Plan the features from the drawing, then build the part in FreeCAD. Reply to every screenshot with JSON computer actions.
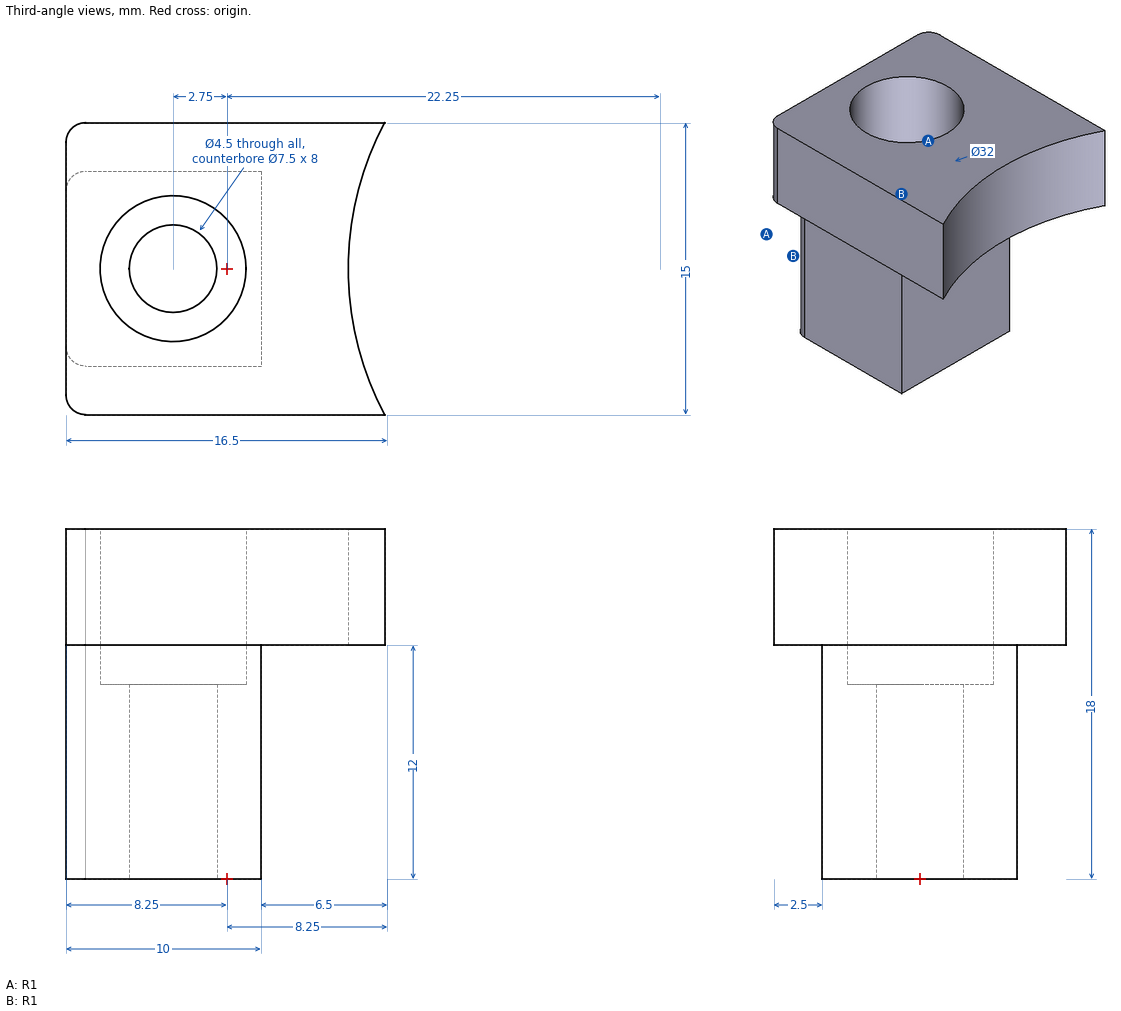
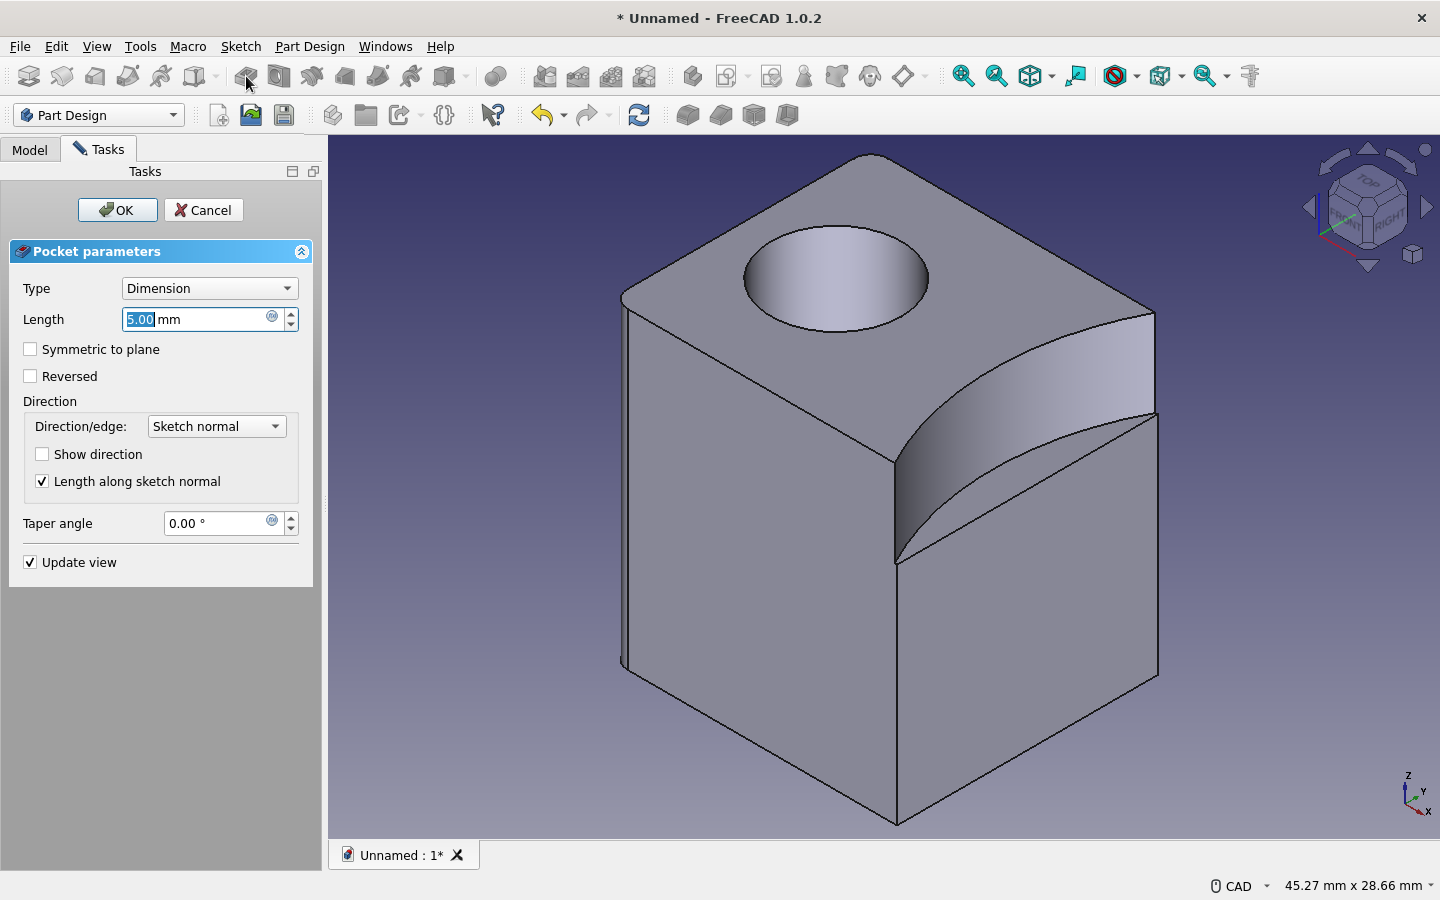
{"action": "left_click", "coordinate": [210, 288]}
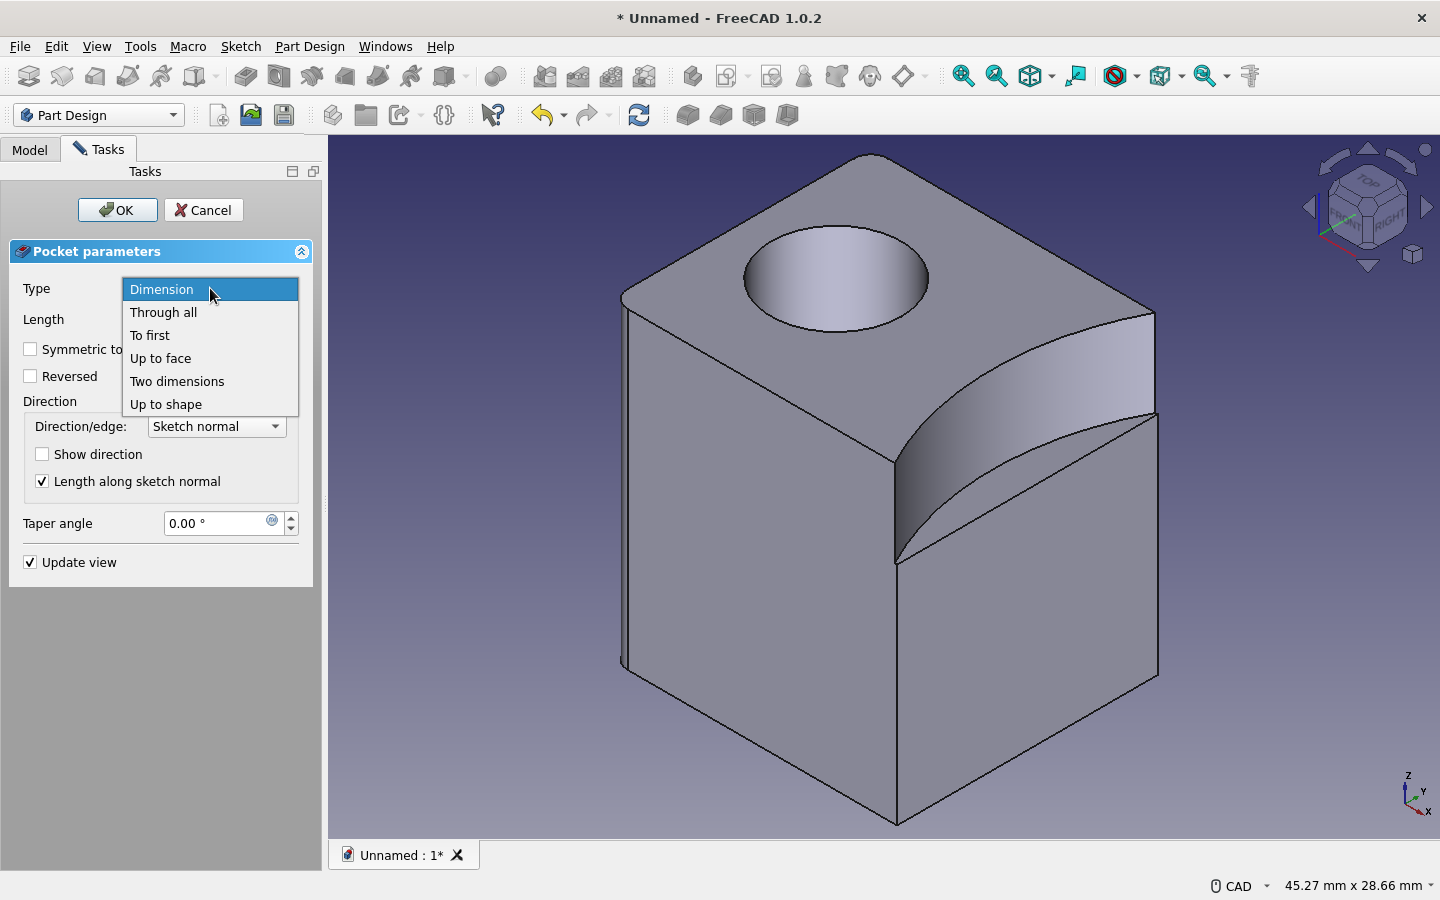
{"action": "left_click", "coordinate": [208, 312]}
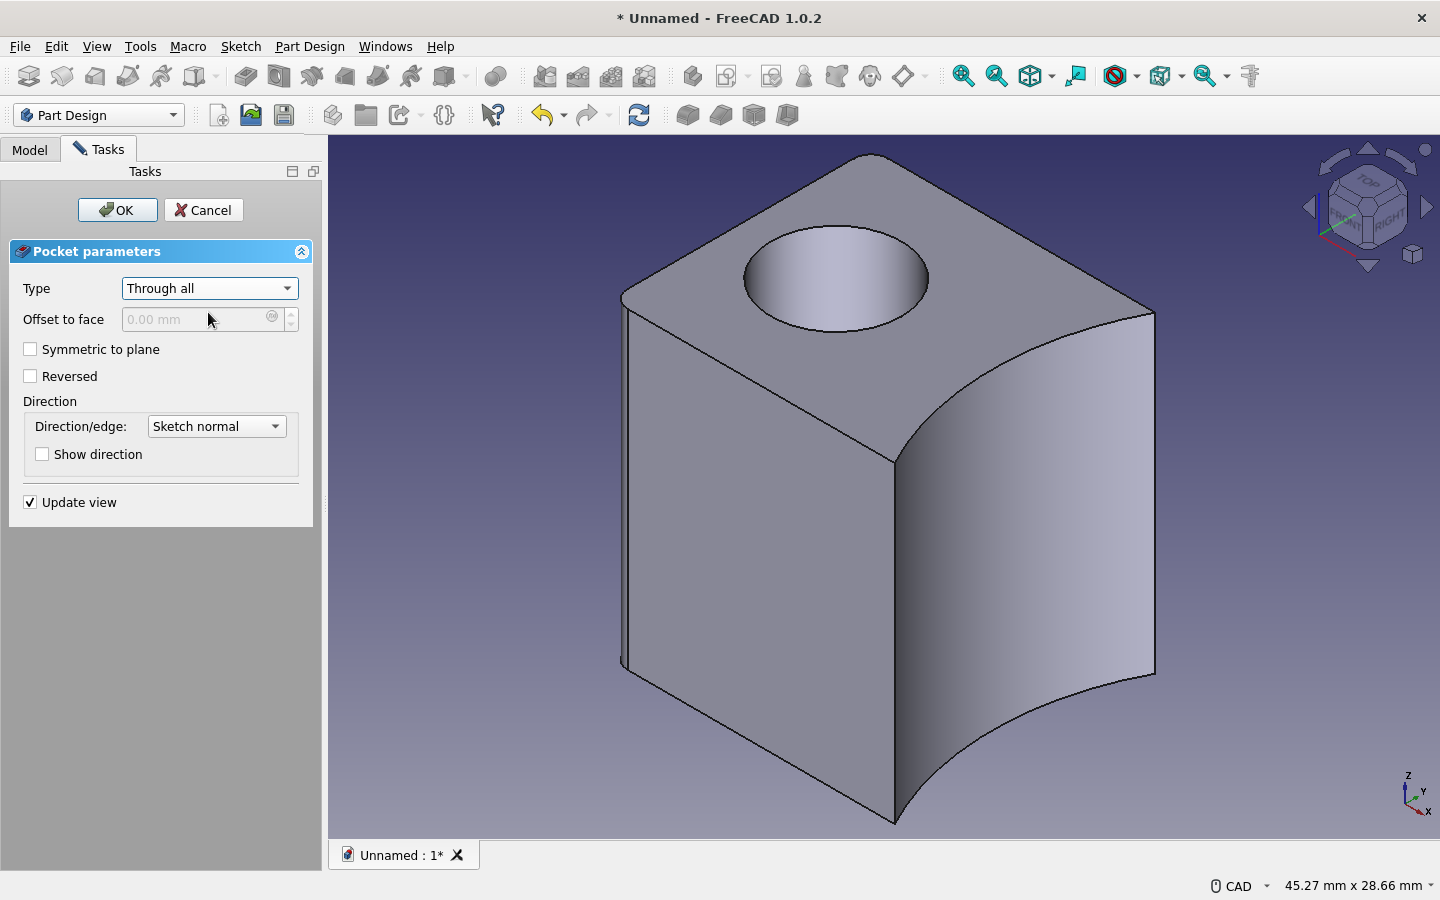
{"action": "left_click", "coordinate": [118, 210]}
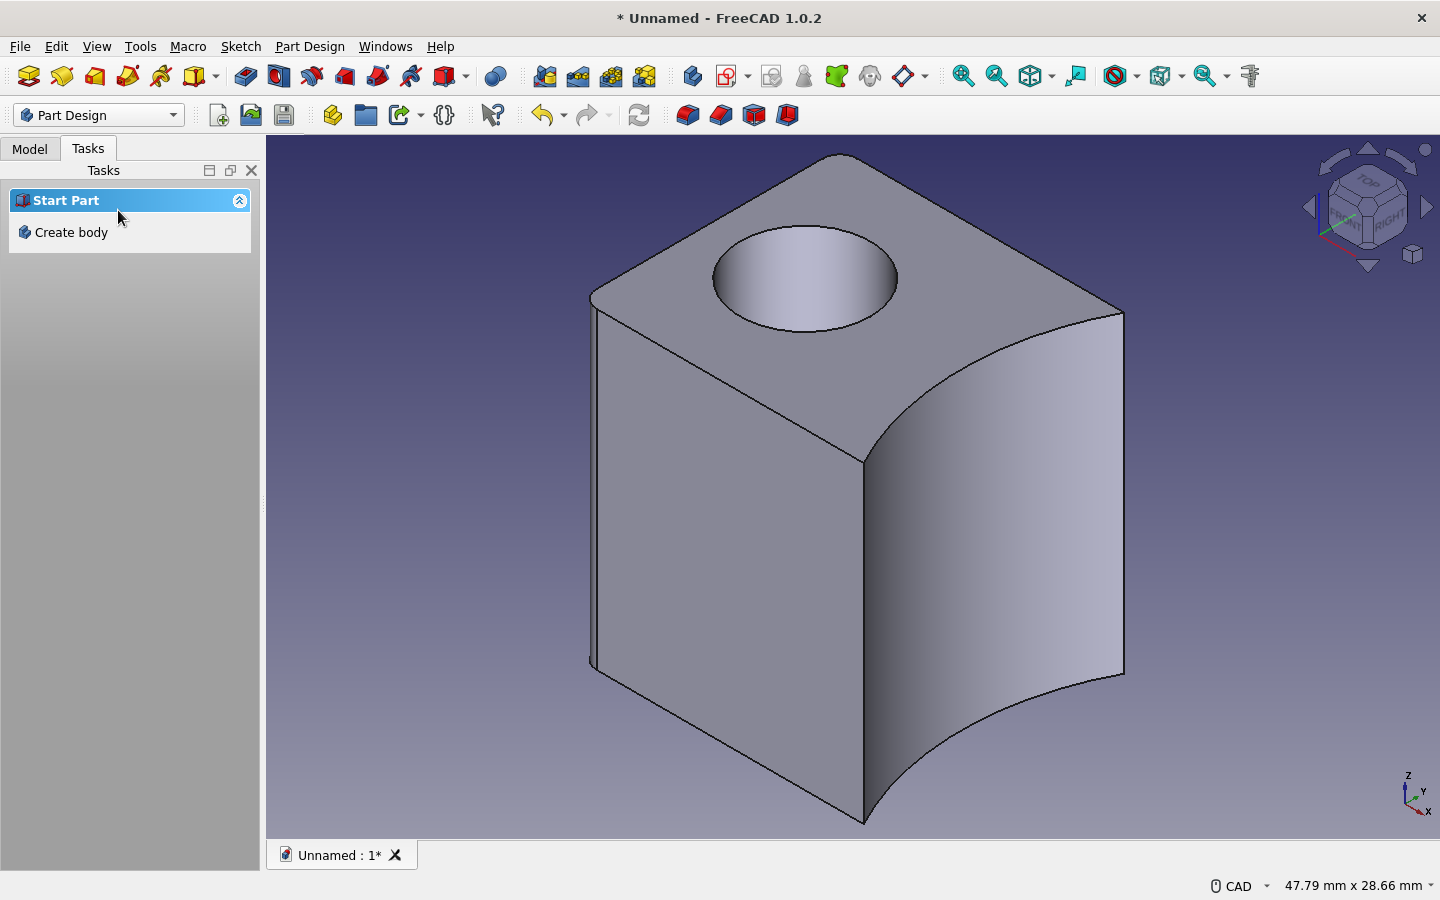
{"action": "key", "text": "4"}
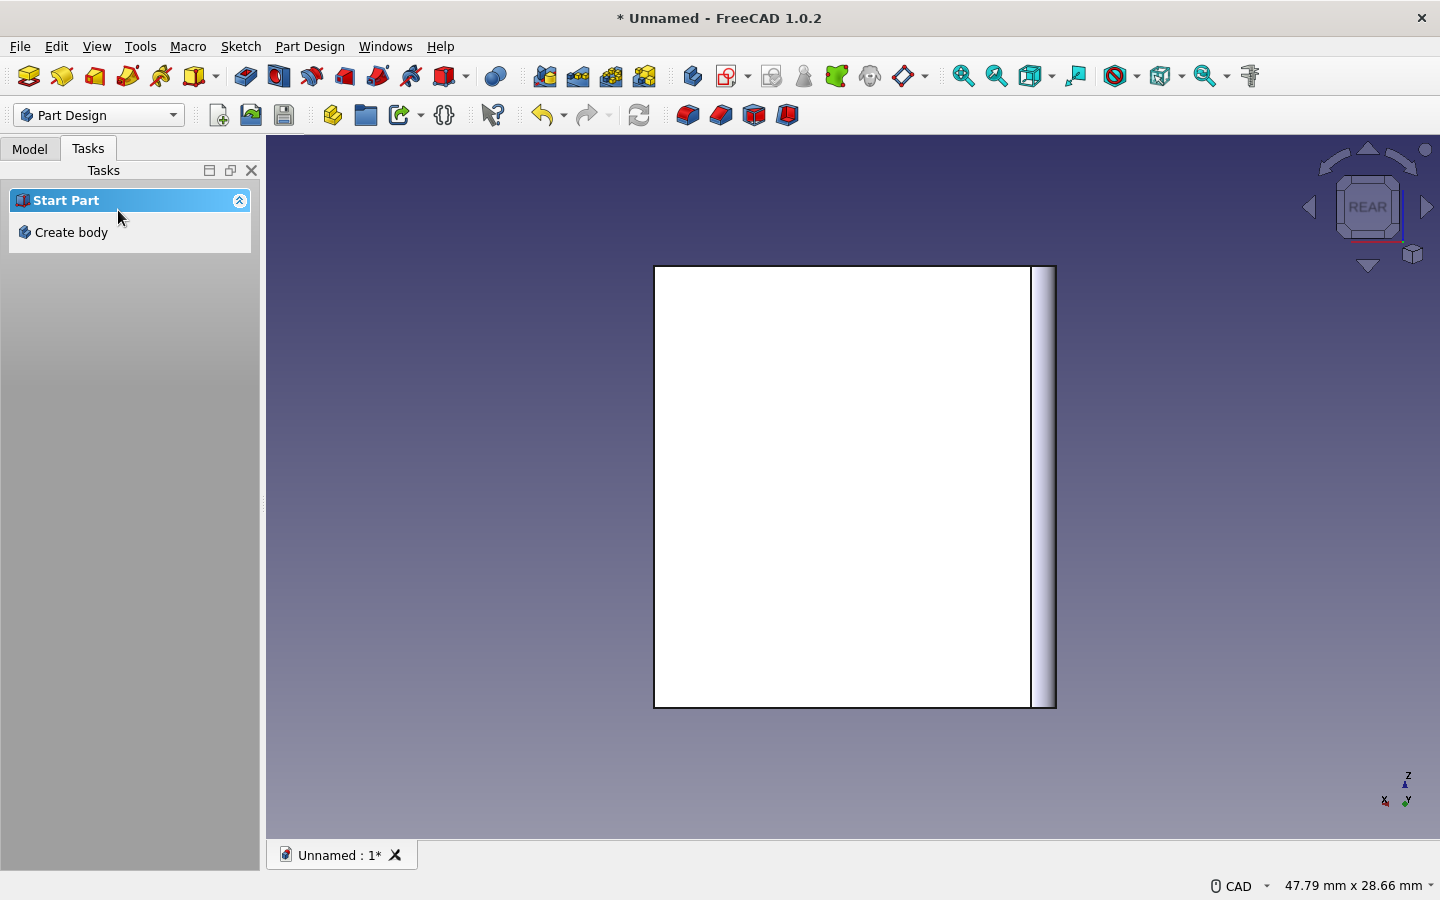
{"action": "left_click", "coordinate": [842, 486]}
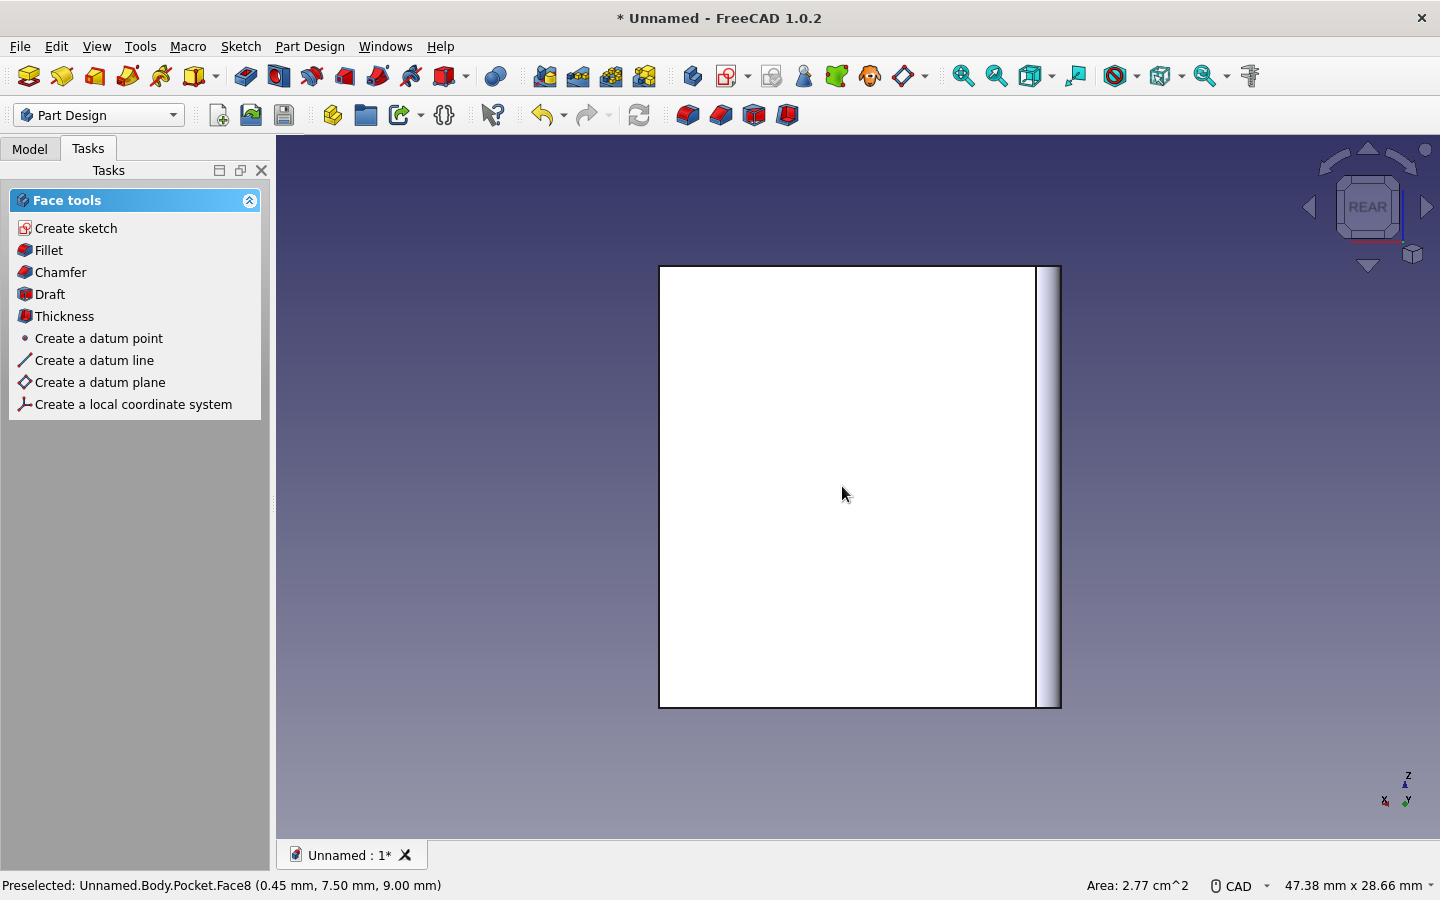
{"action": "left_click", "coordinate": [726, 76]}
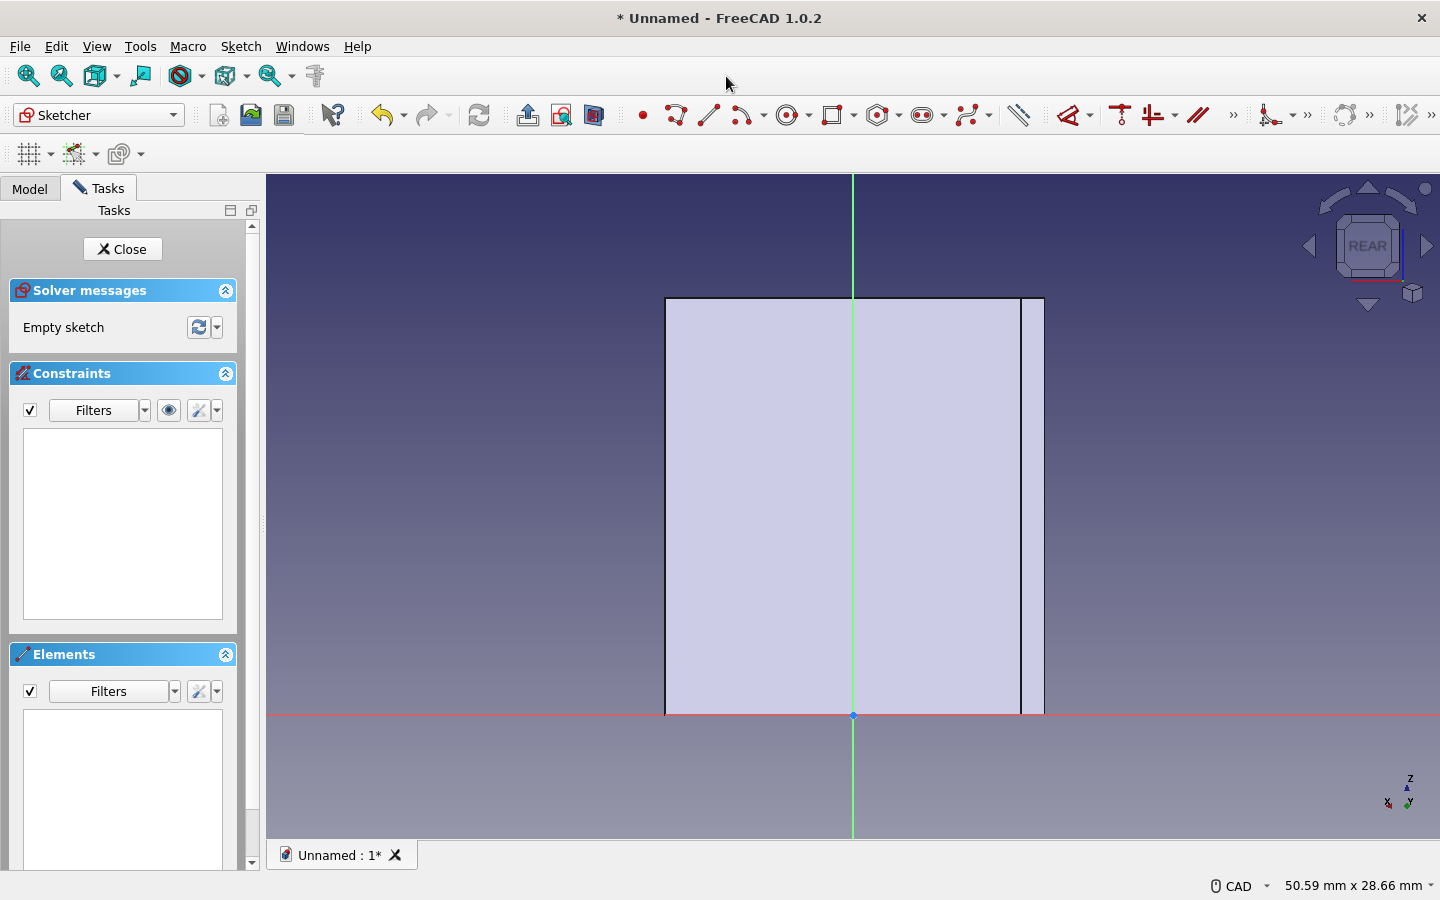
{"action": "scroll", "coordinate": [702, 718], "scroll_direction": "up", "scroll_amount": 2}